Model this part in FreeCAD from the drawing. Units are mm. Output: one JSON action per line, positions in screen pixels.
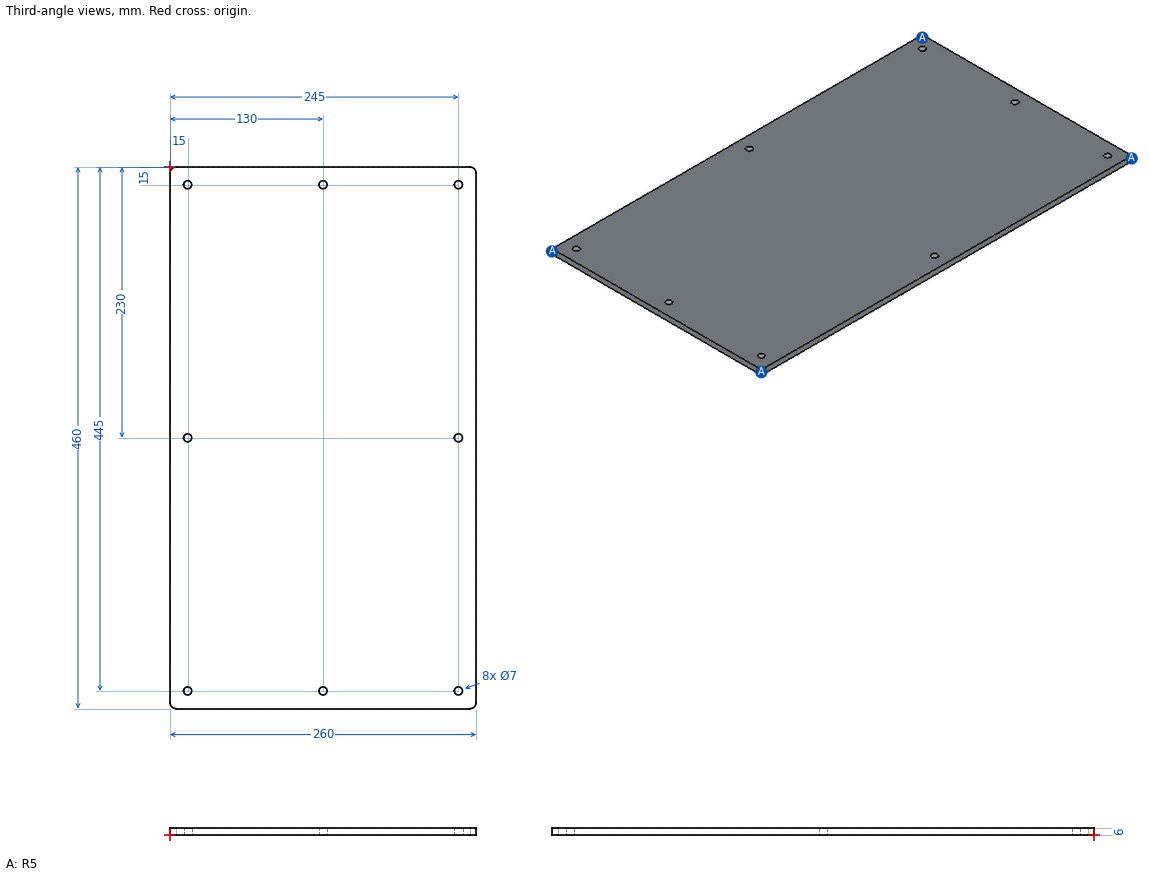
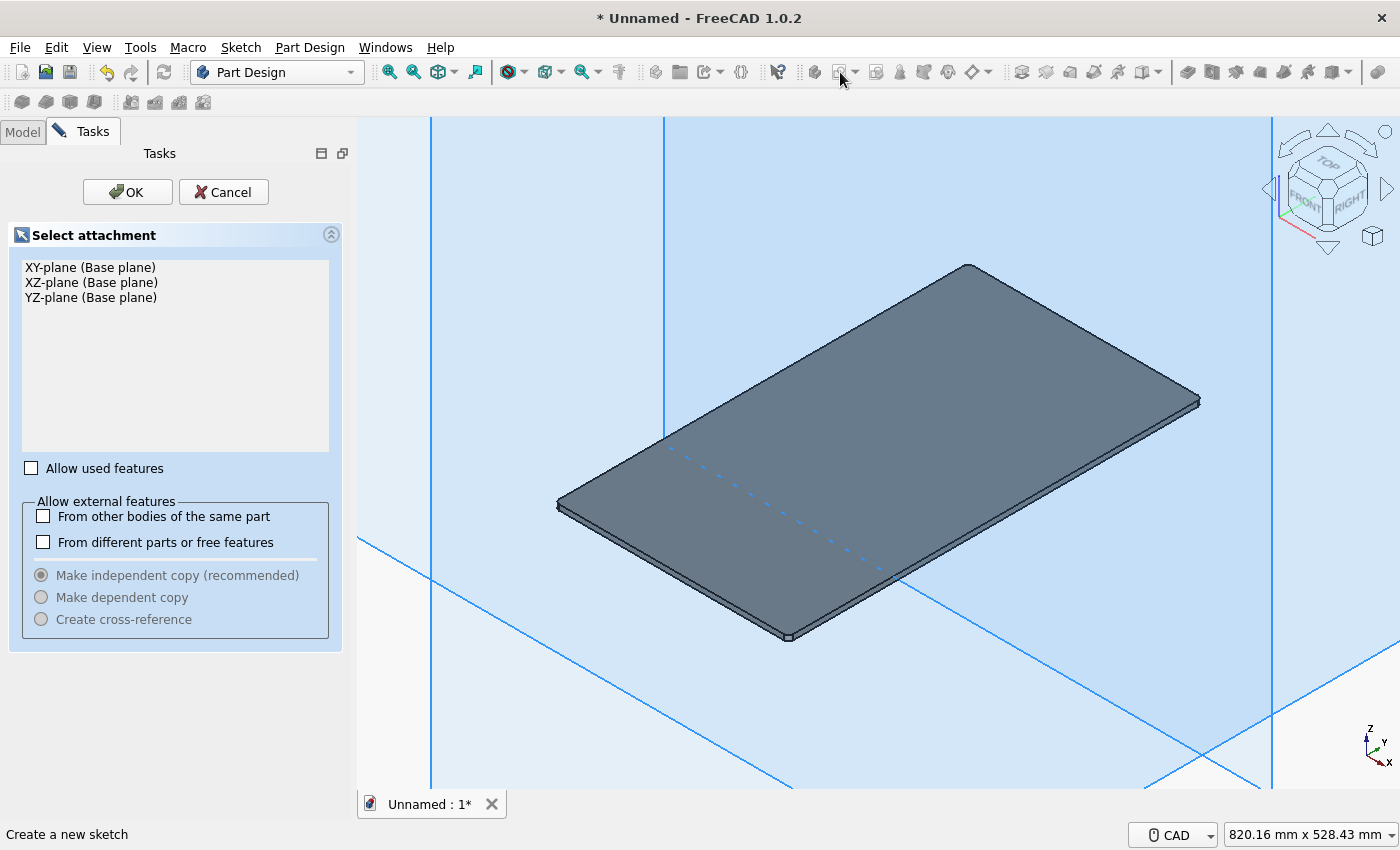
{"action": "left_click", "coordinate": [82, 268]}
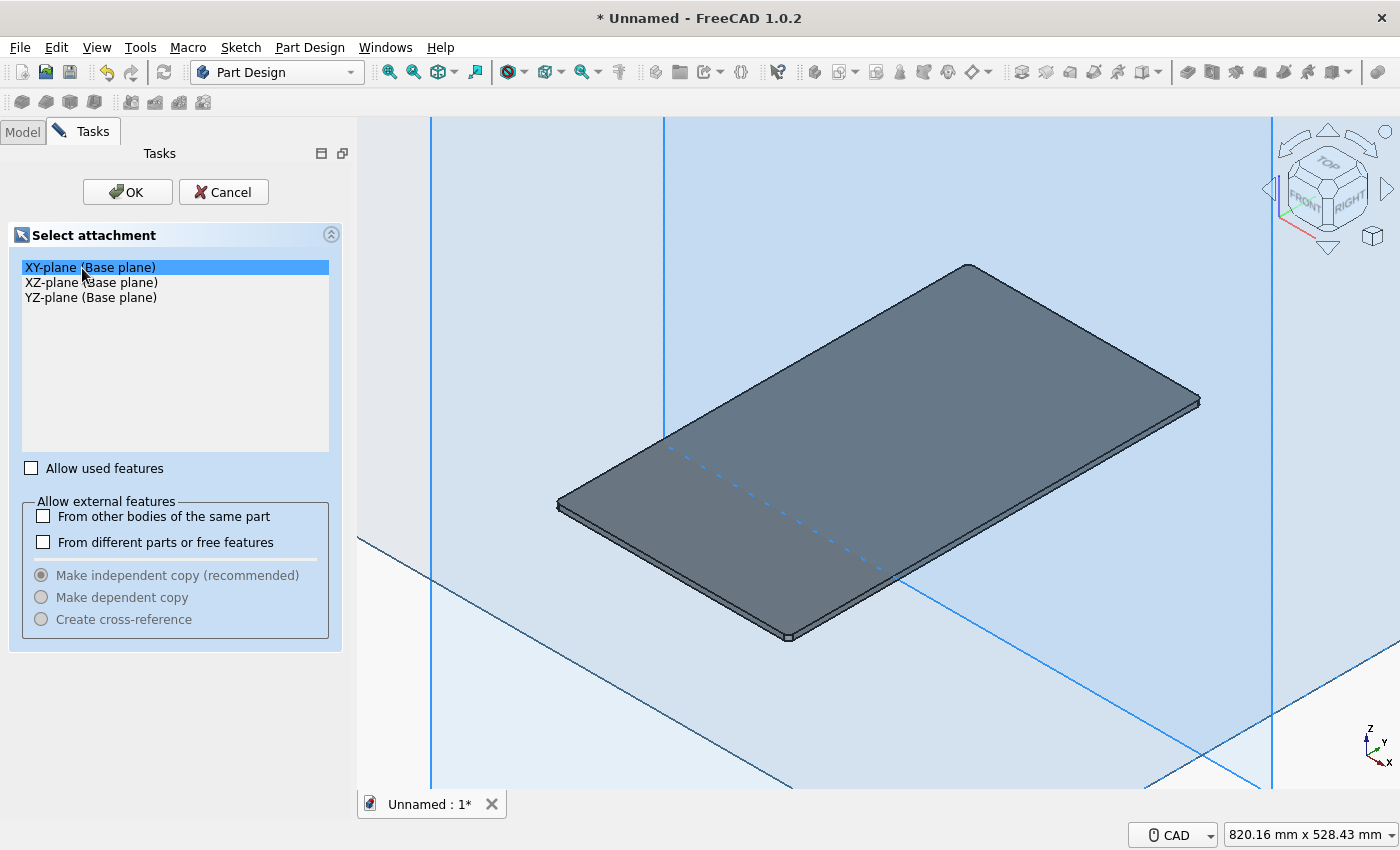
{"action": "left_click", "coordinate": [128, 192]}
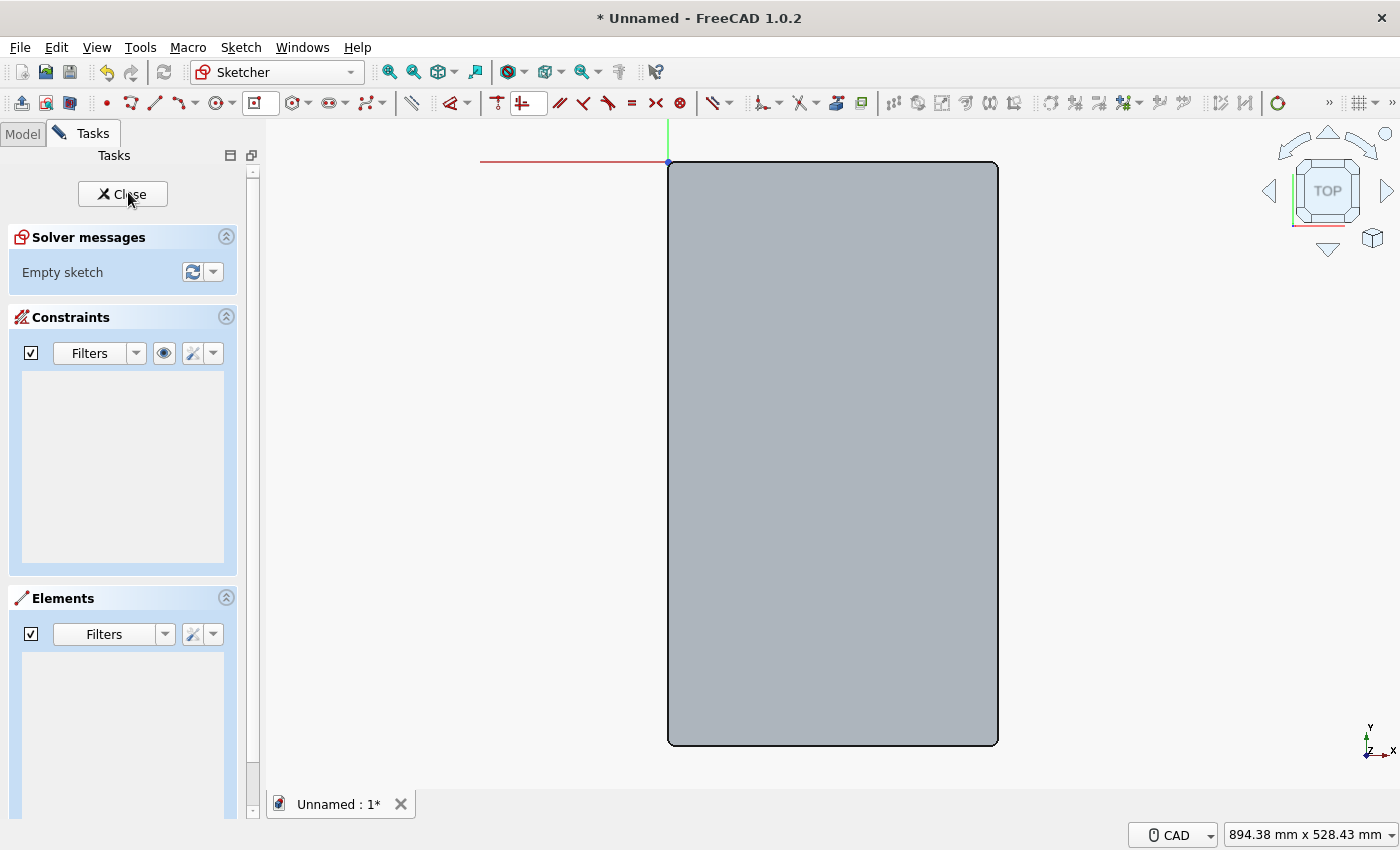
{"action": "key", "text": "q s"}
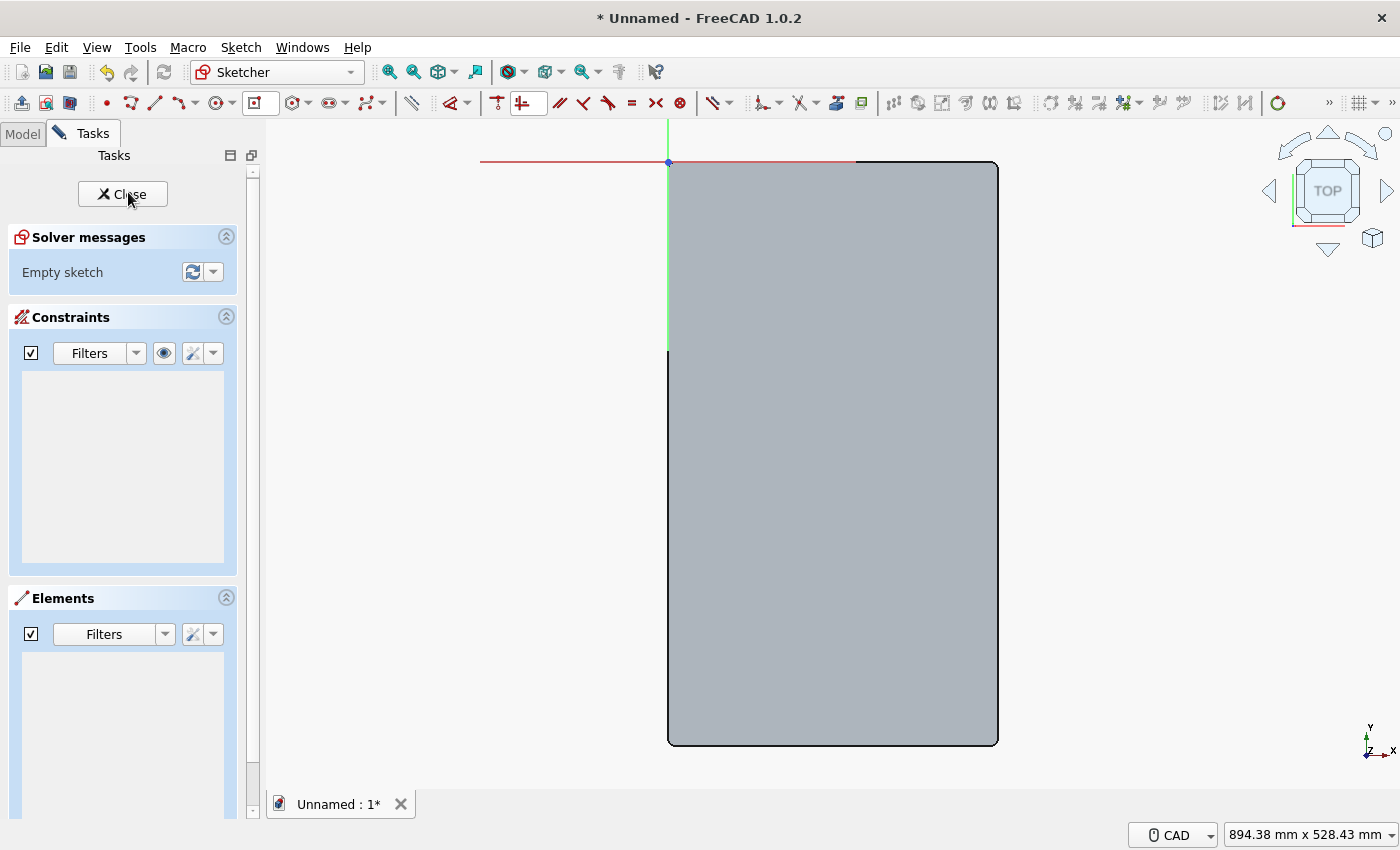
{"action": "scroll", "coordinate": [488, 487], "scroll_direction": "down", "scroll_amount": 1}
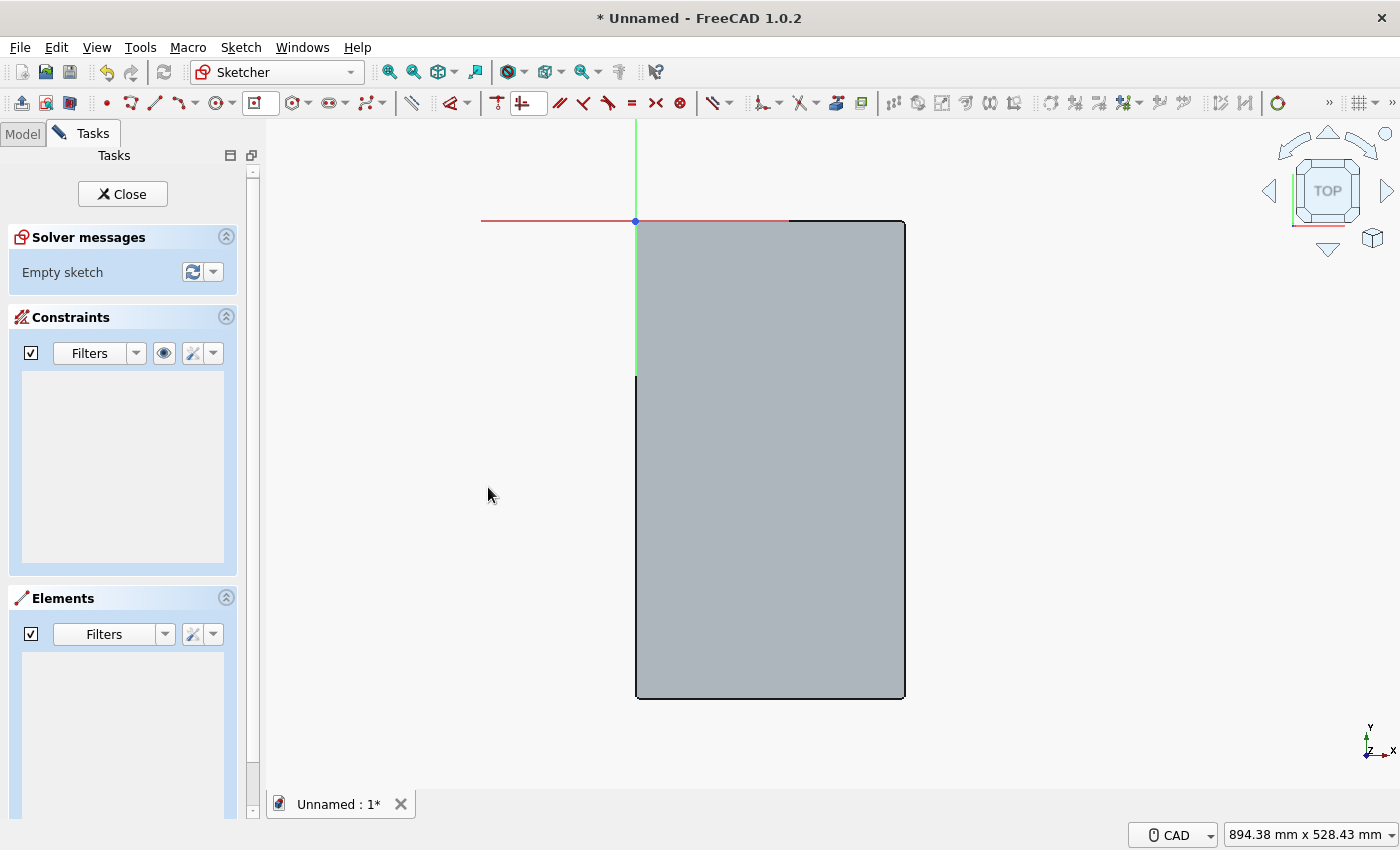
{"action": "key", "text": "g c"}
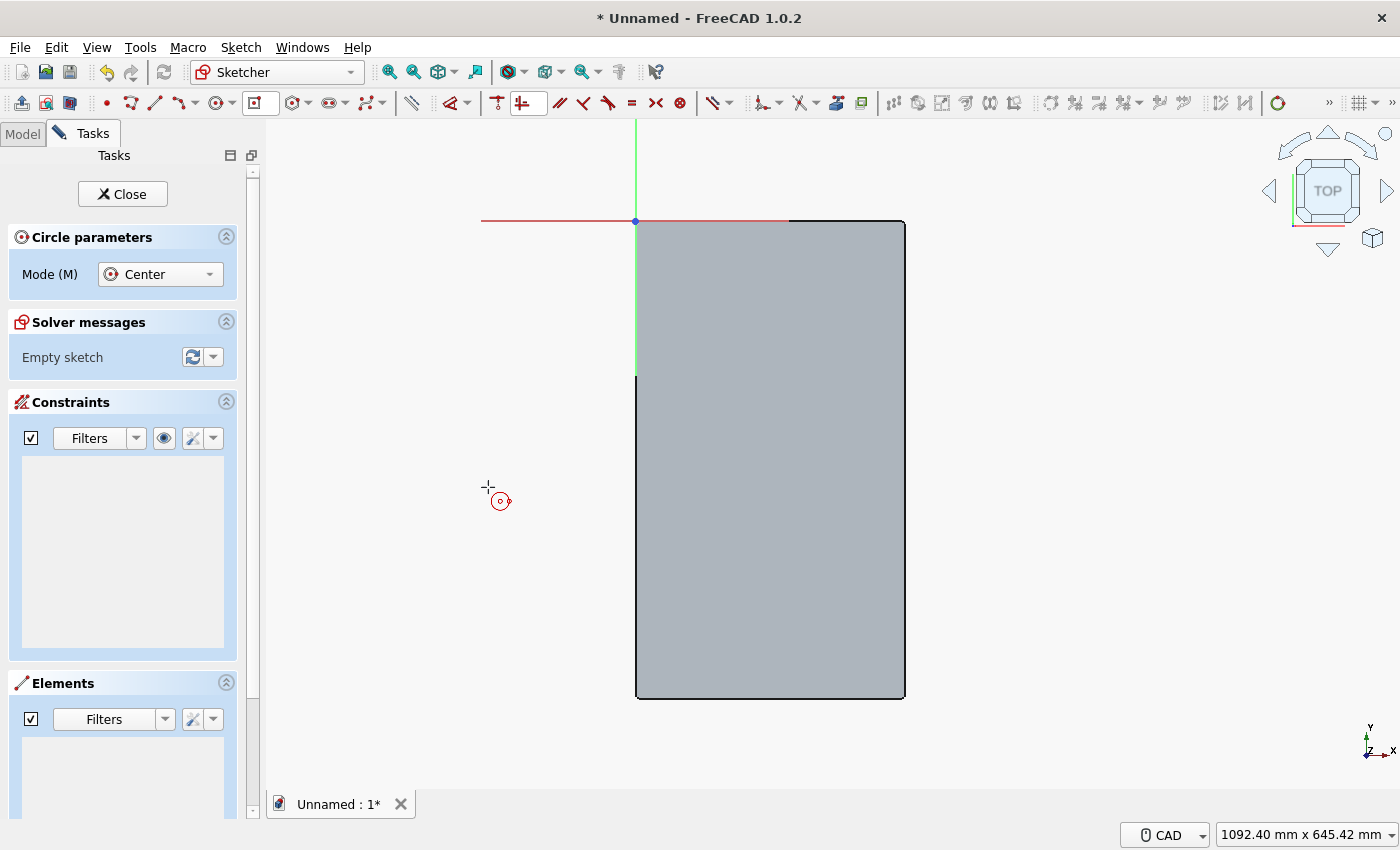
{"action": "scroll", "coordinate": [890, 683], "scroll_direction": "up", "scroll_amount": 10}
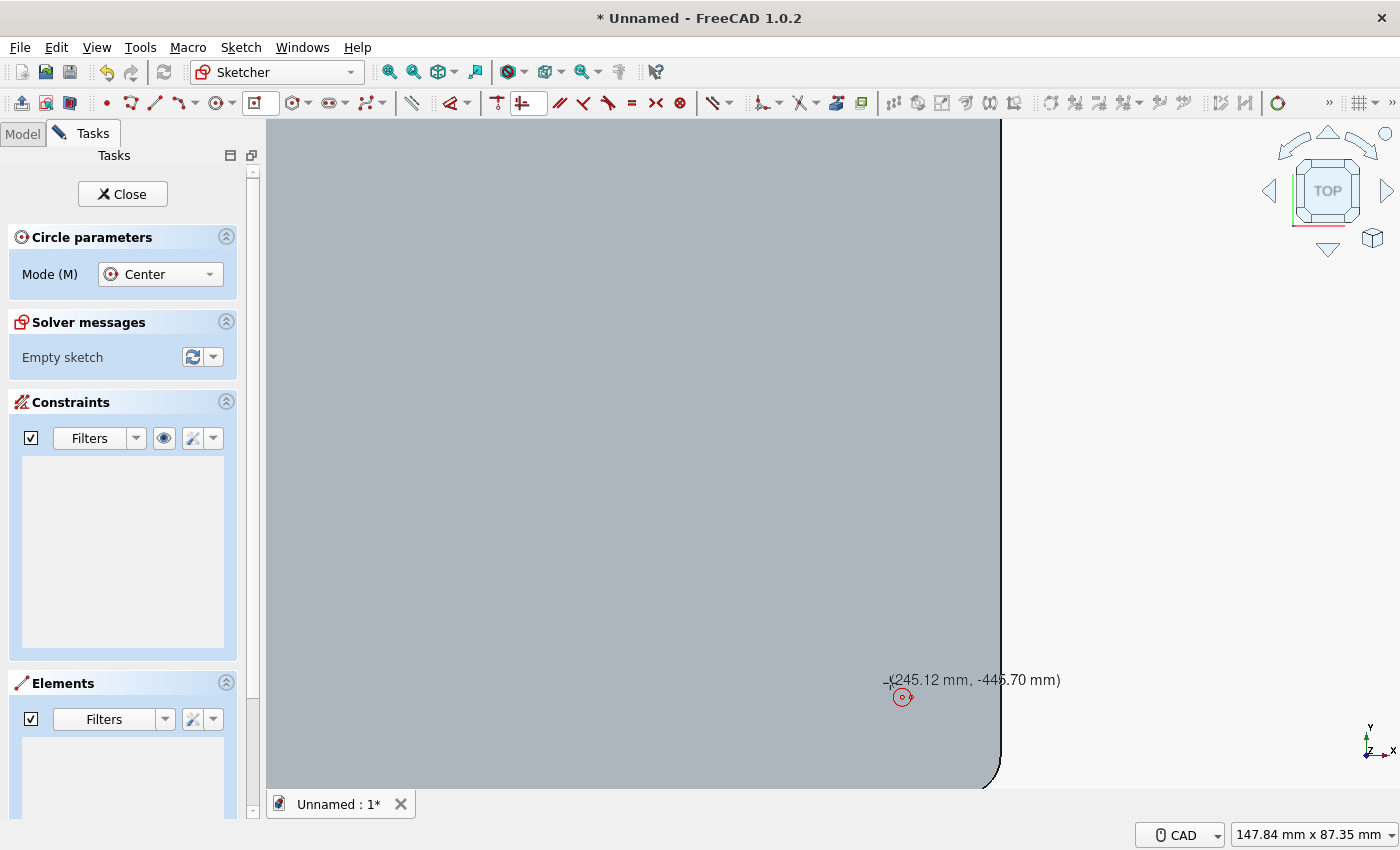
{"action": "scroll", "coordinate": [891, 684], "scroll_direction": "down", "scroll_amount": 10}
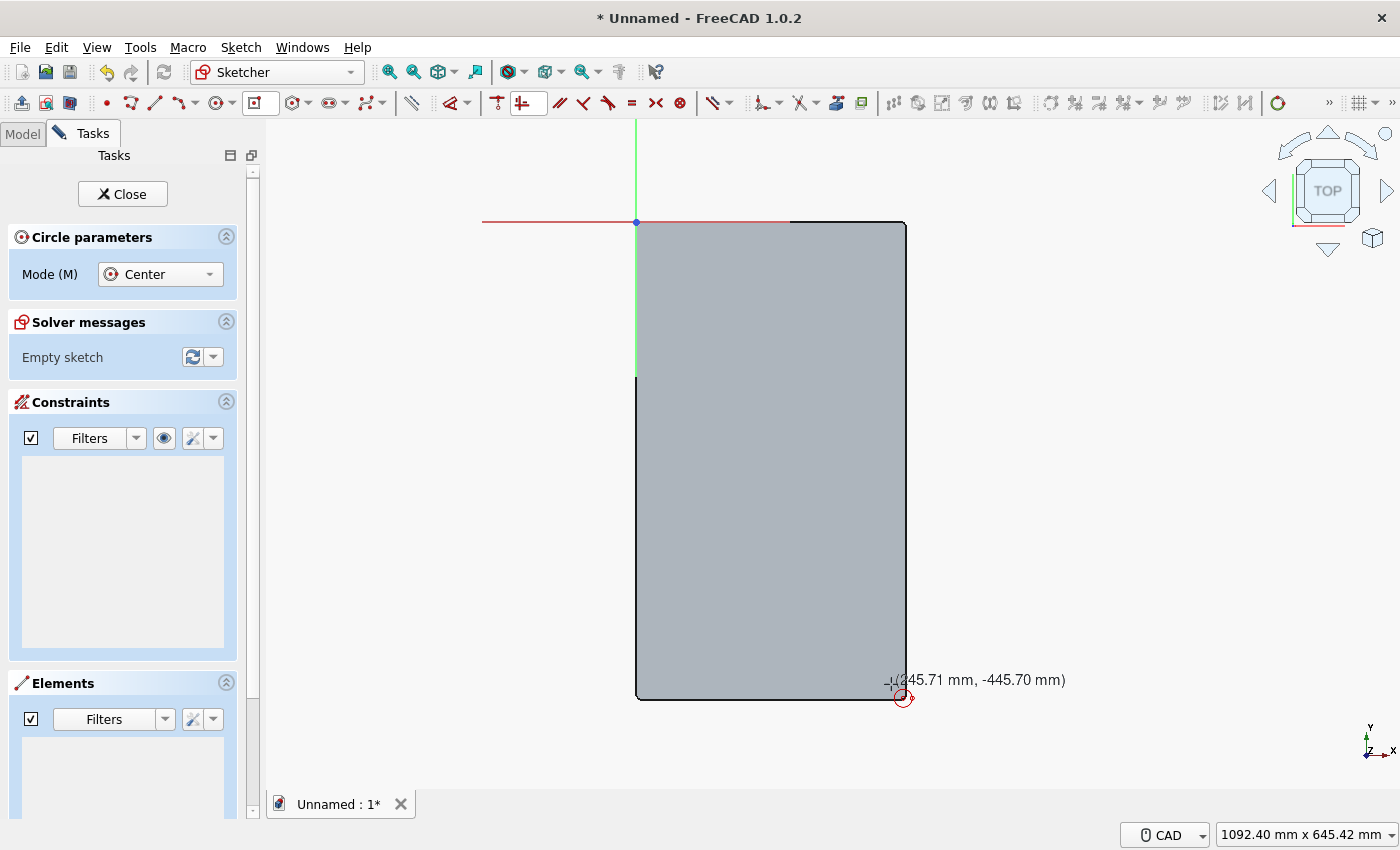
{"action": "left_click", "coordinate": [891, 684]}